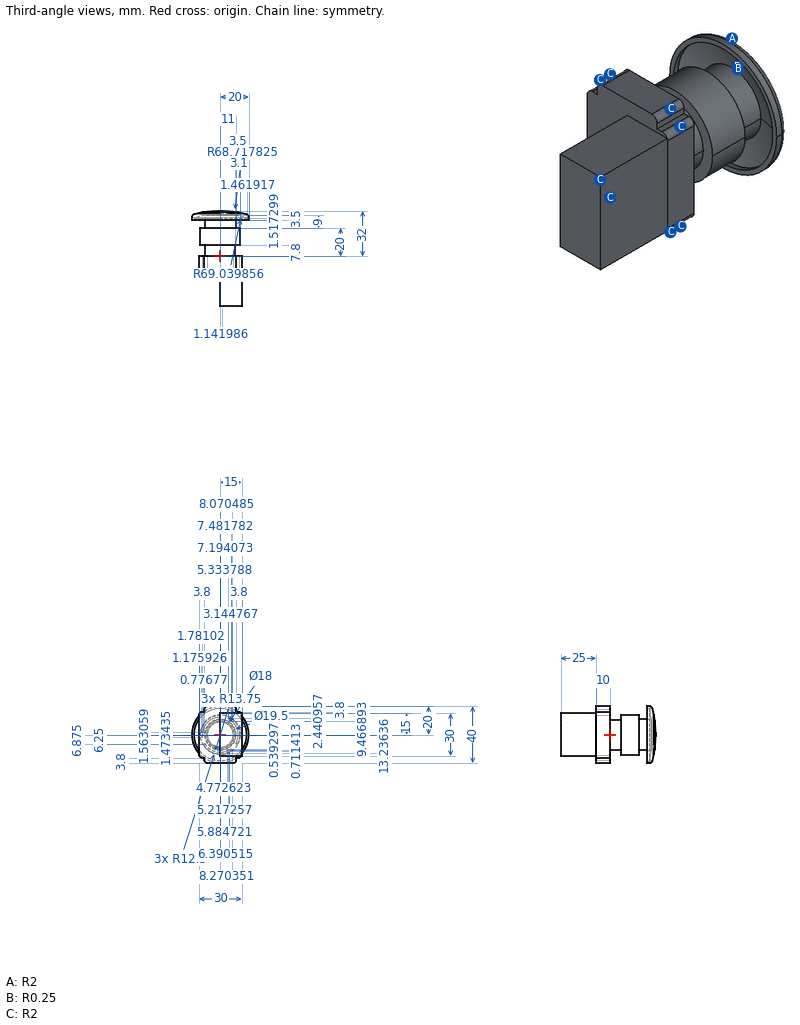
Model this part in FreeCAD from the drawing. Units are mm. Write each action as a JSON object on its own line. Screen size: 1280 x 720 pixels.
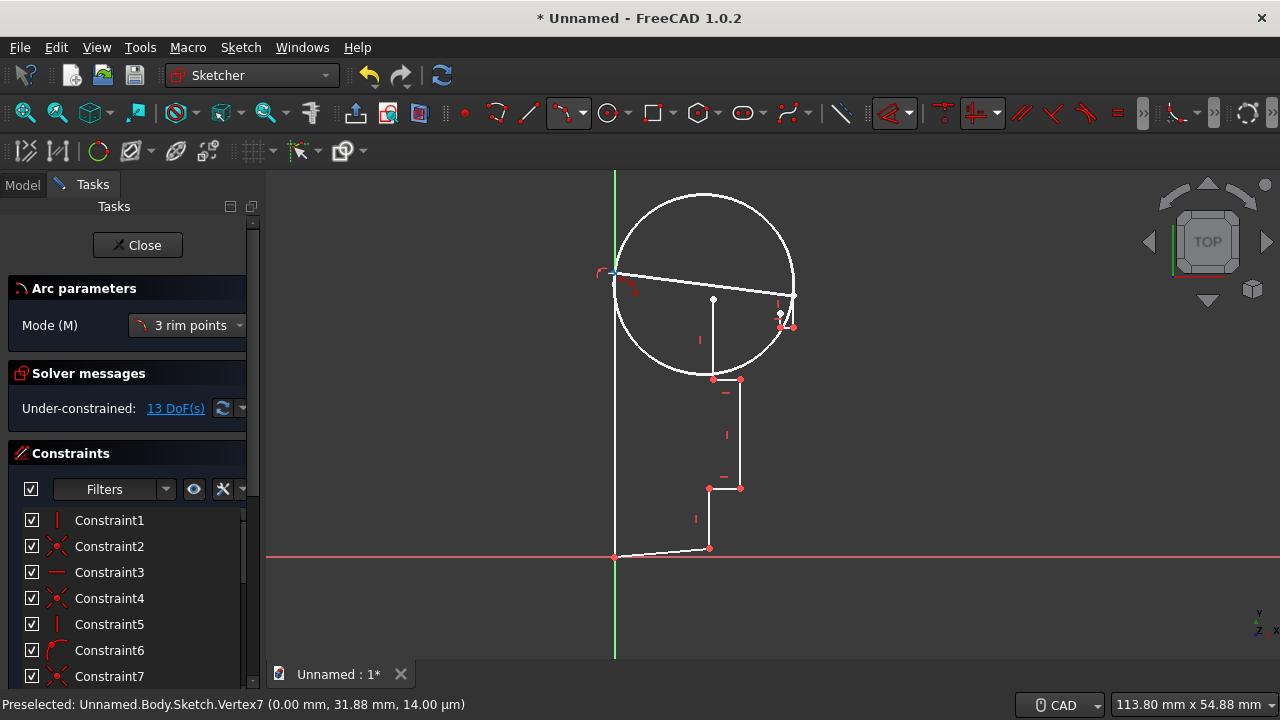
{"action": "scroll", "coordinate": [705, 277], "scroll_direction": "up", "scroll_amount": 5}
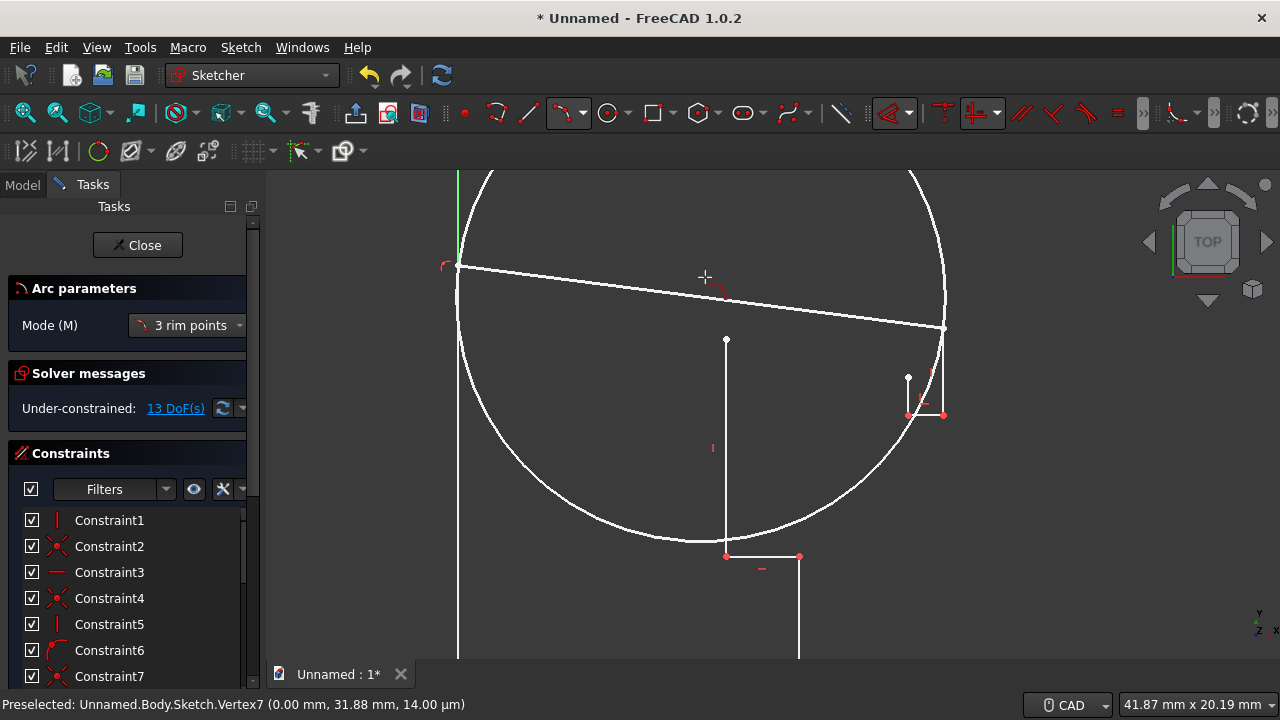
{"action": "left_click", "coordinate": [703, 277]}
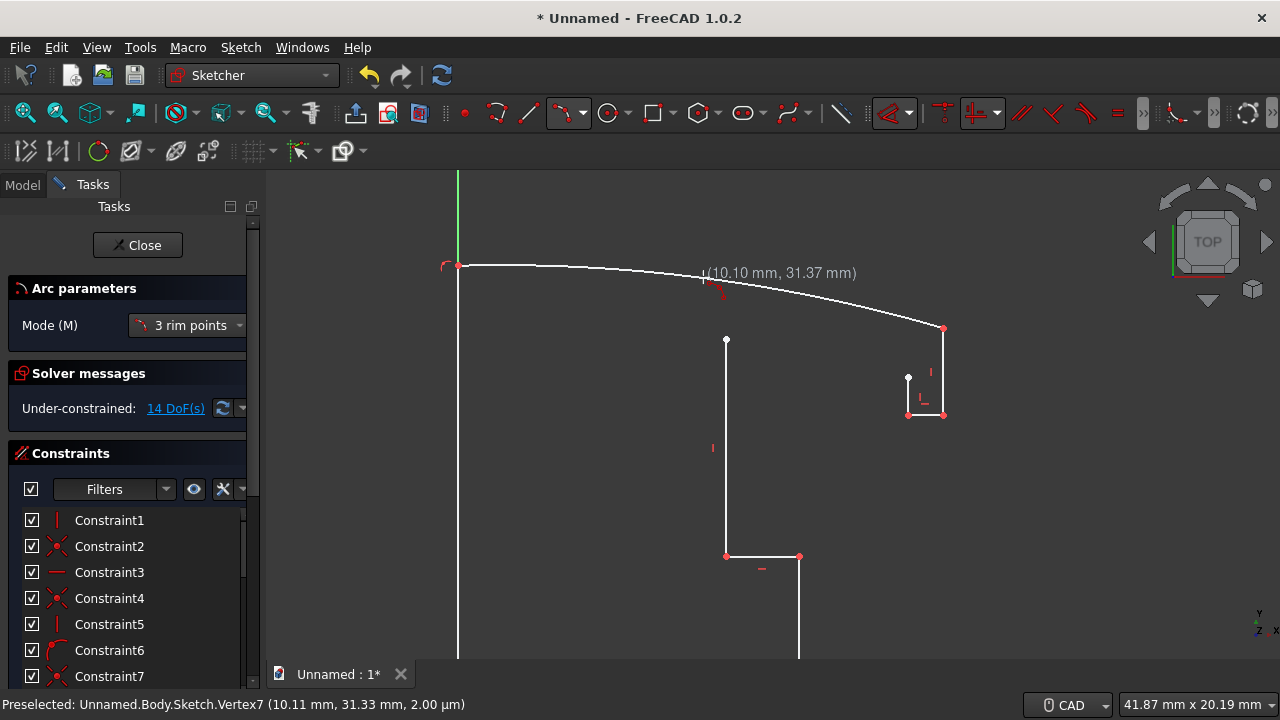
{"action": "left_click", "coordinate": [726, 339]}
{"action": "left_click", "coordinate": [908, 377]}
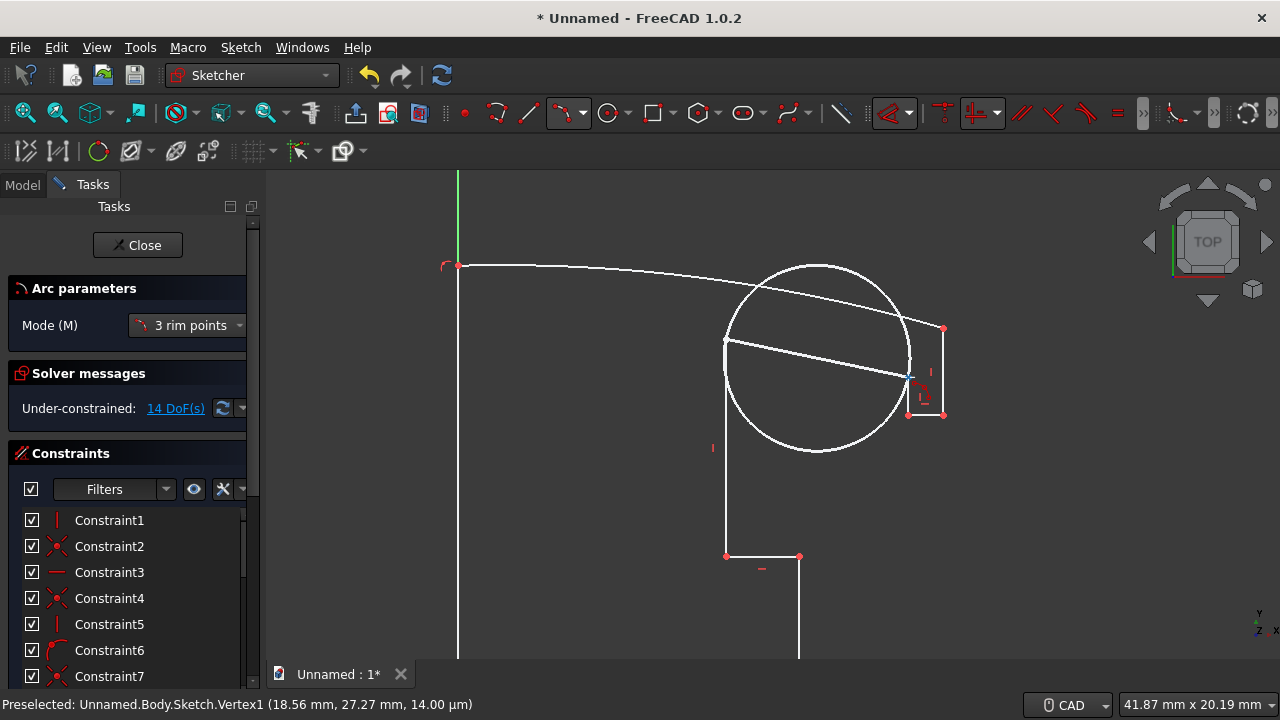
{"action": "scroll", "coordinate": [817, 352], "scroll_direction": "up", "scroll_amount": 10}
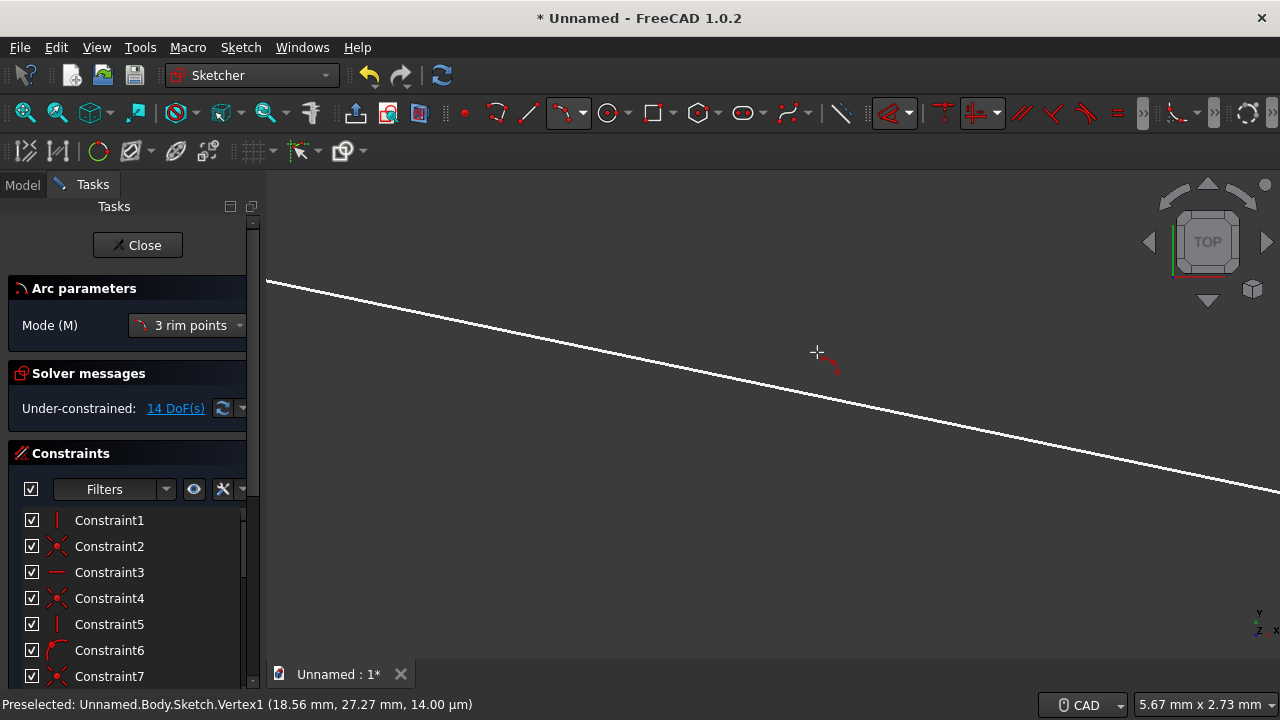
{"action": "left_click", "coordinate": [812, 352]}
{"action": "key", "text": "Escape"}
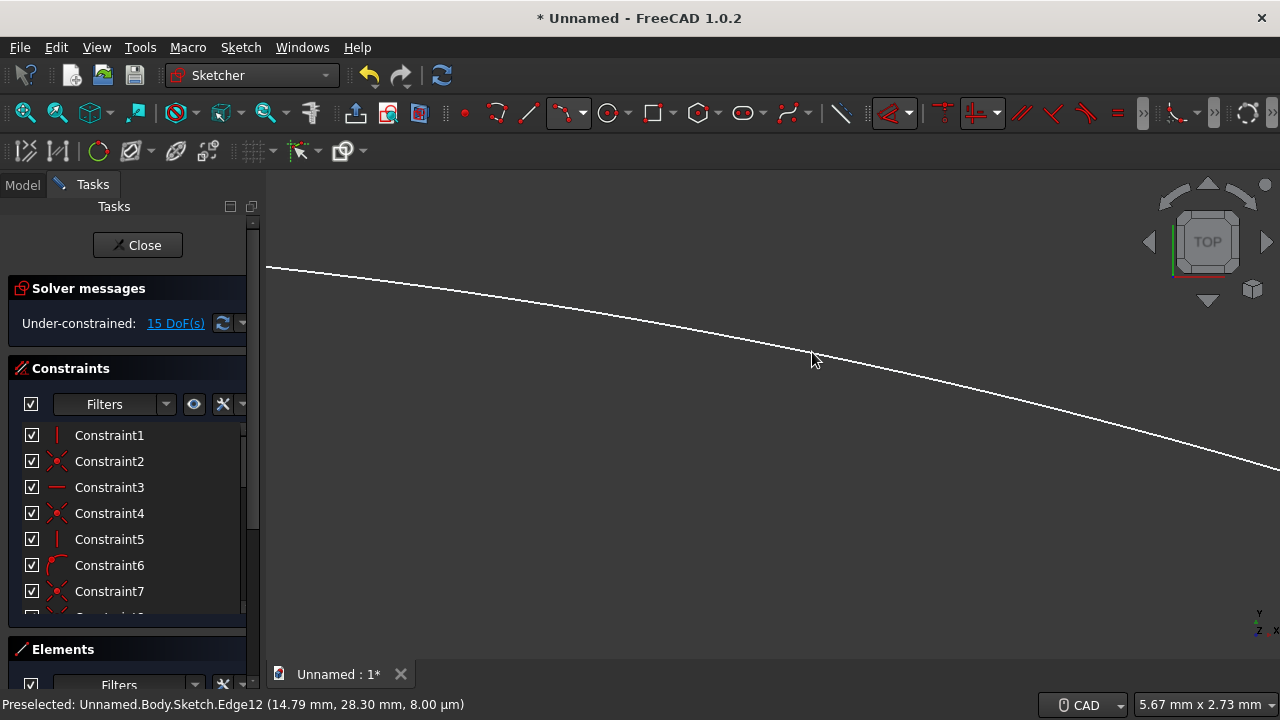
{"action": "scroll", "coordinate": [744, 302], "scroll_direction": "down", "scroll_amount": 15}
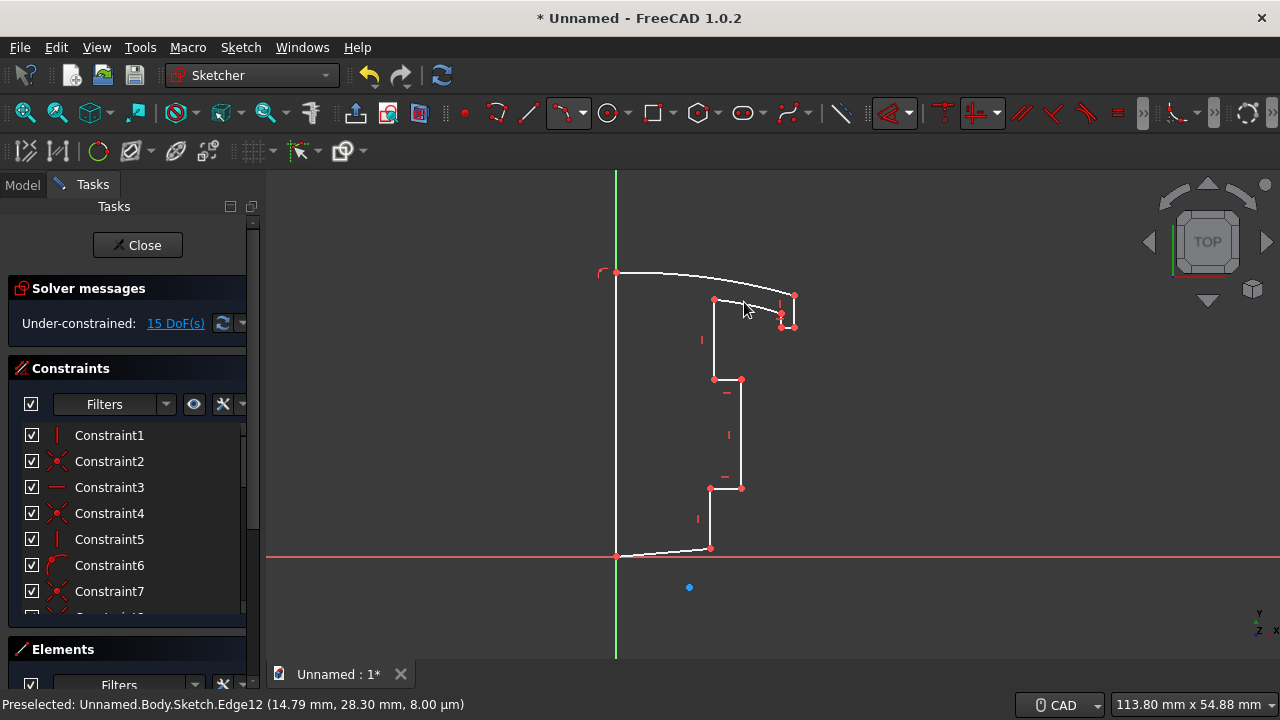
{"action": "scroll", "coordinate": [644, 555], "scroll_direction": "up", "scroll_amount": 9}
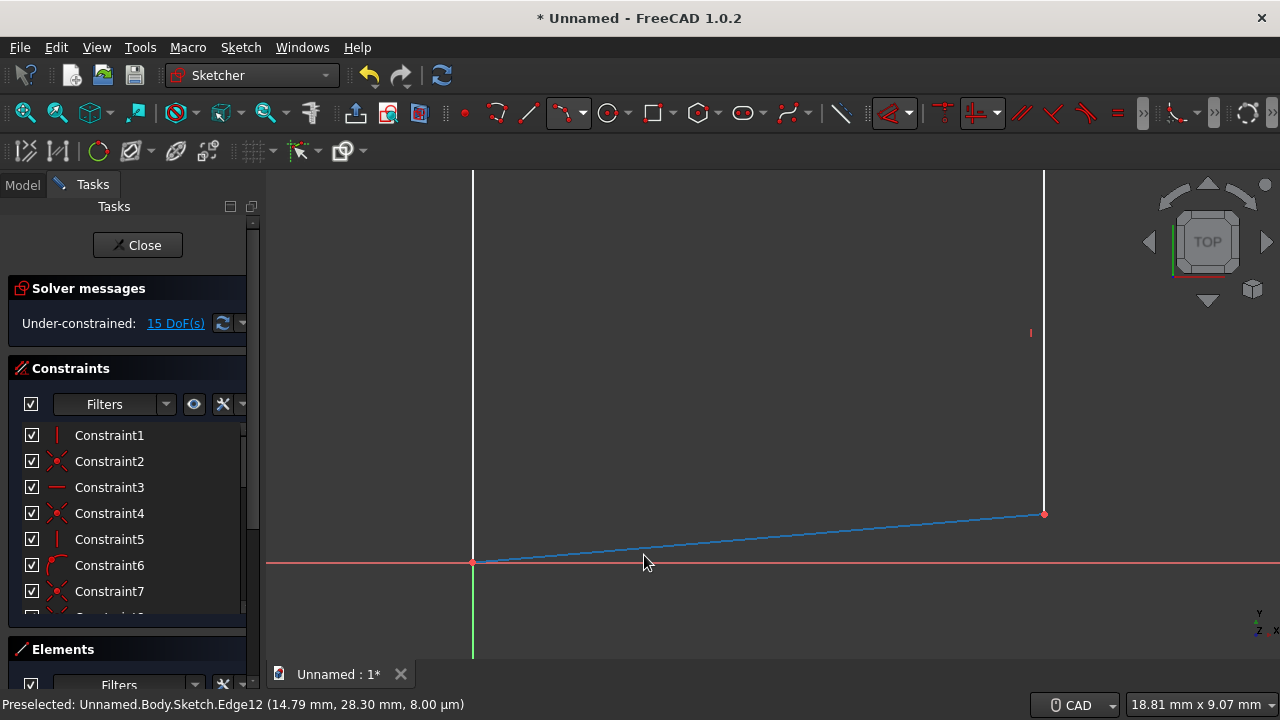
{"action": "left_click", "coordinate": [644, 548]}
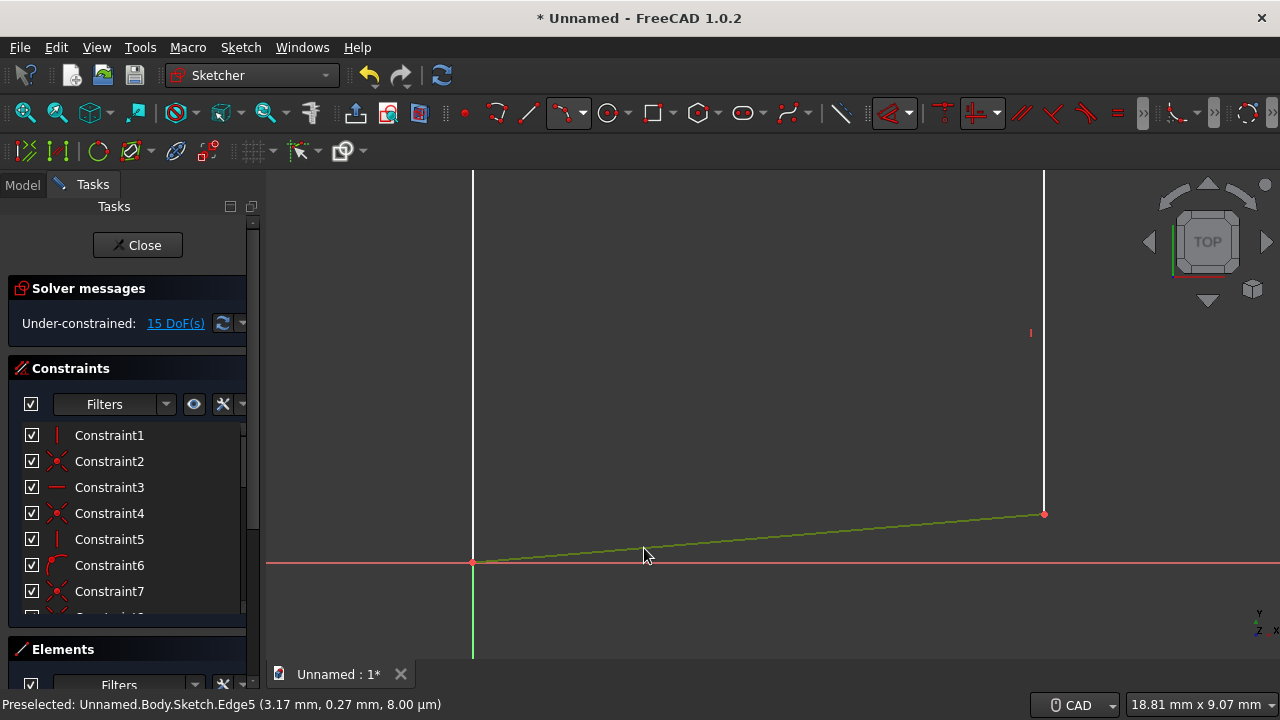
{"action": "left_click", "coordinate": [1000, 114]}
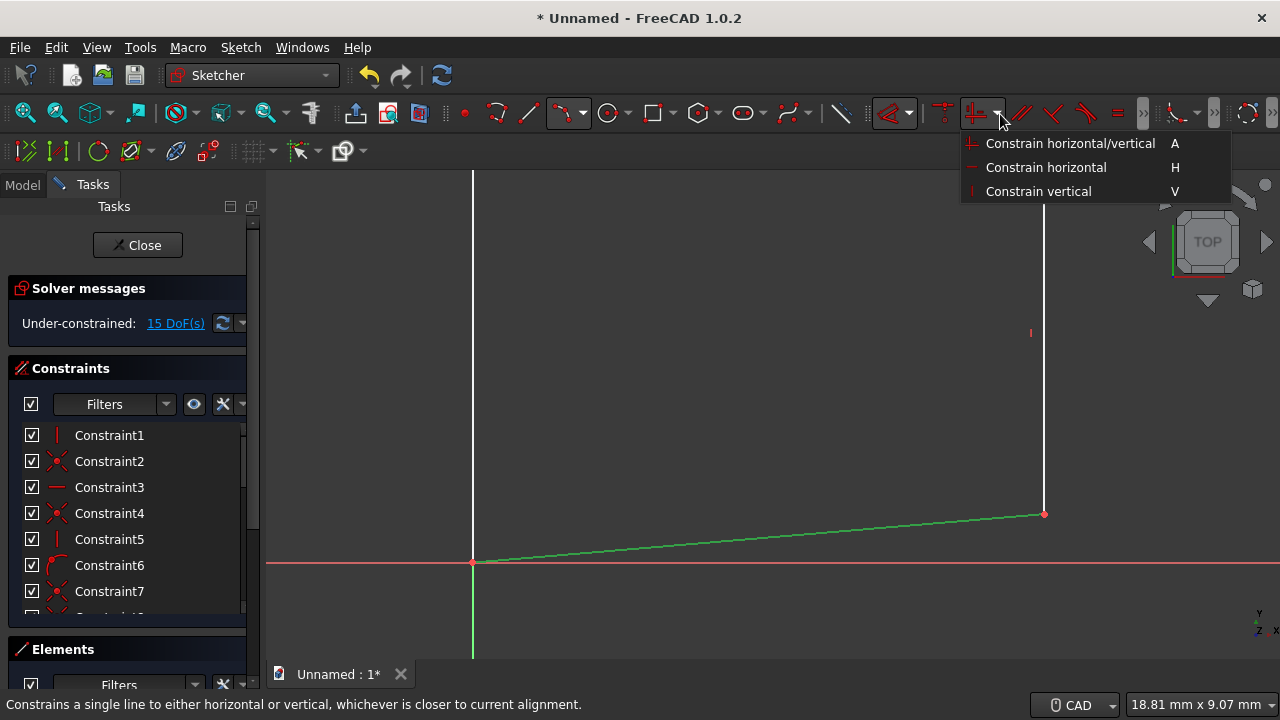
{"action": "left_click", "coordinate": [1096, 167]}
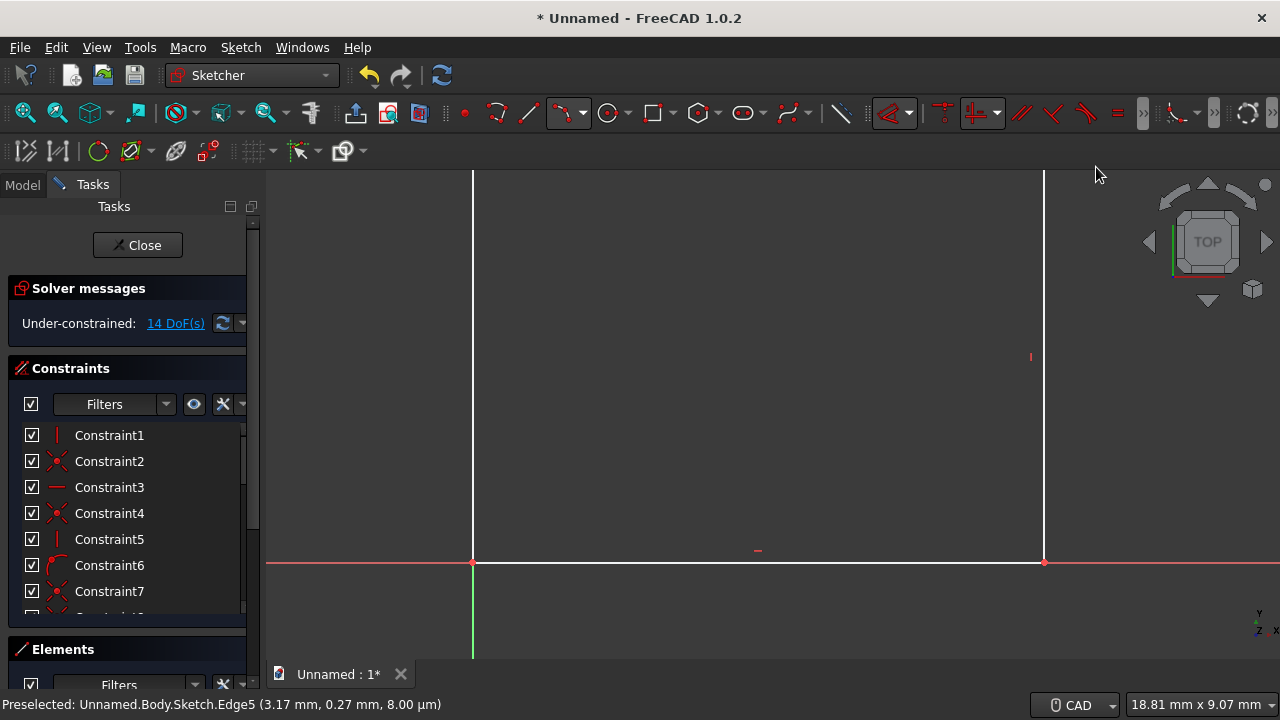
{"action": "left_click", "coordinate": [888, 114]}